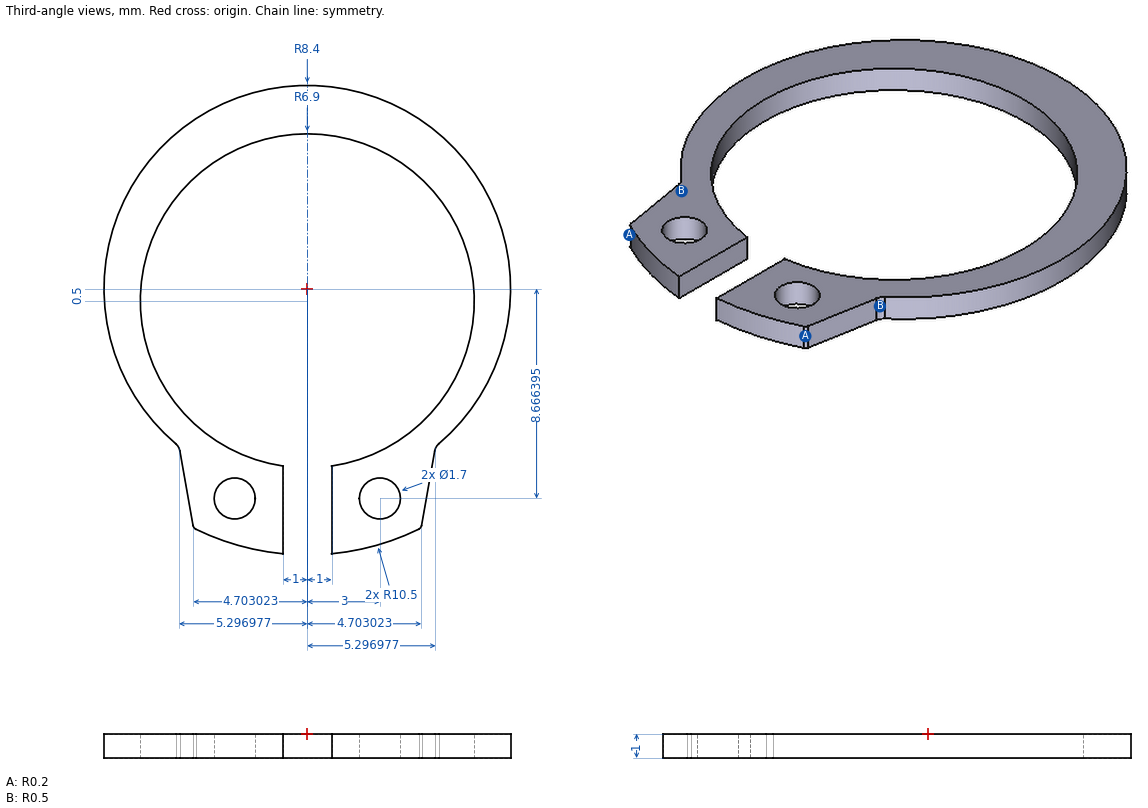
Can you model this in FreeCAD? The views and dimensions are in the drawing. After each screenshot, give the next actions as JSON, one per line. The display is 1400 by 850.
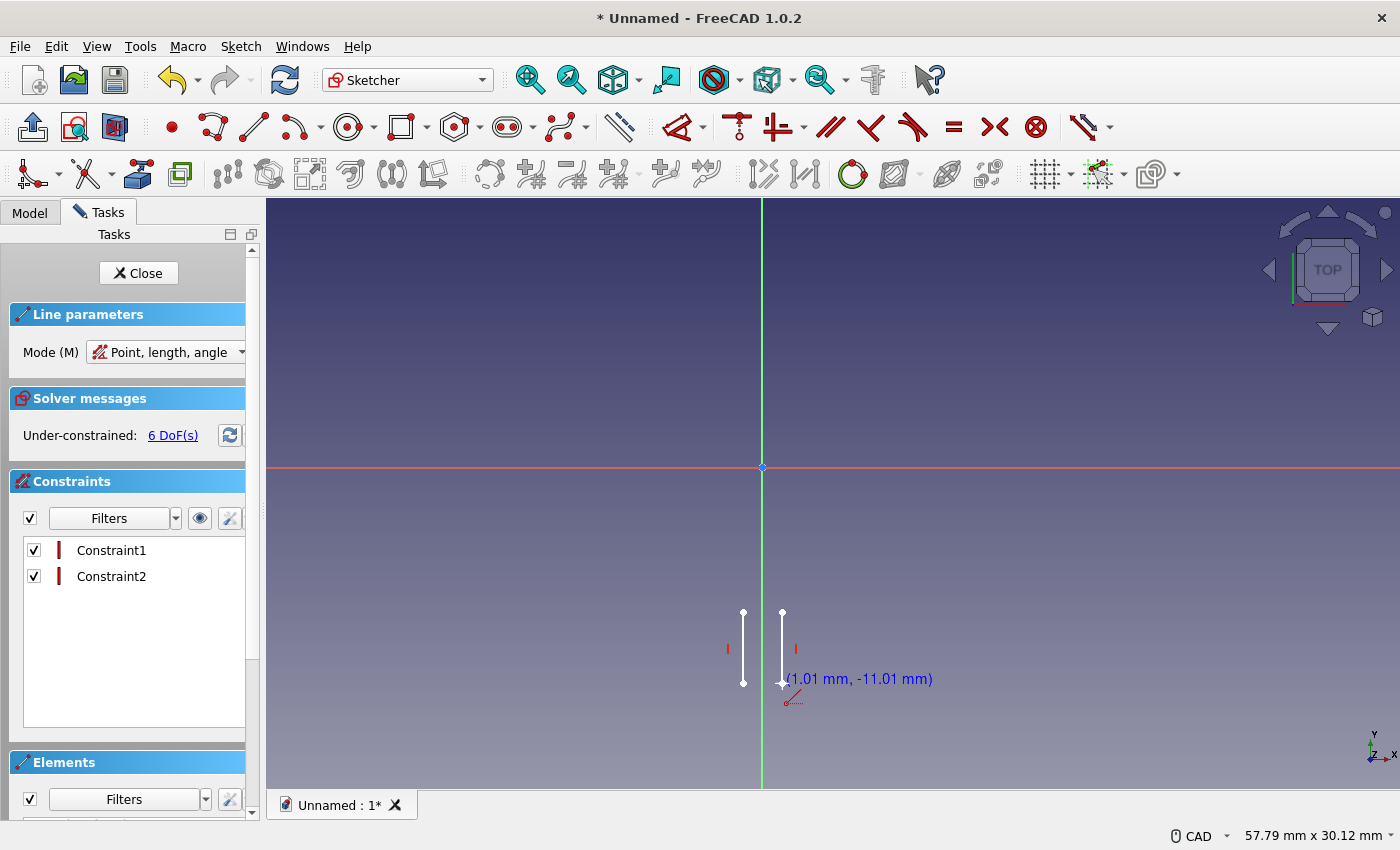
{"action": "left_click", "coordinate": [854, 662]}
{"action": "left_click", "coordinate": [866, 596]}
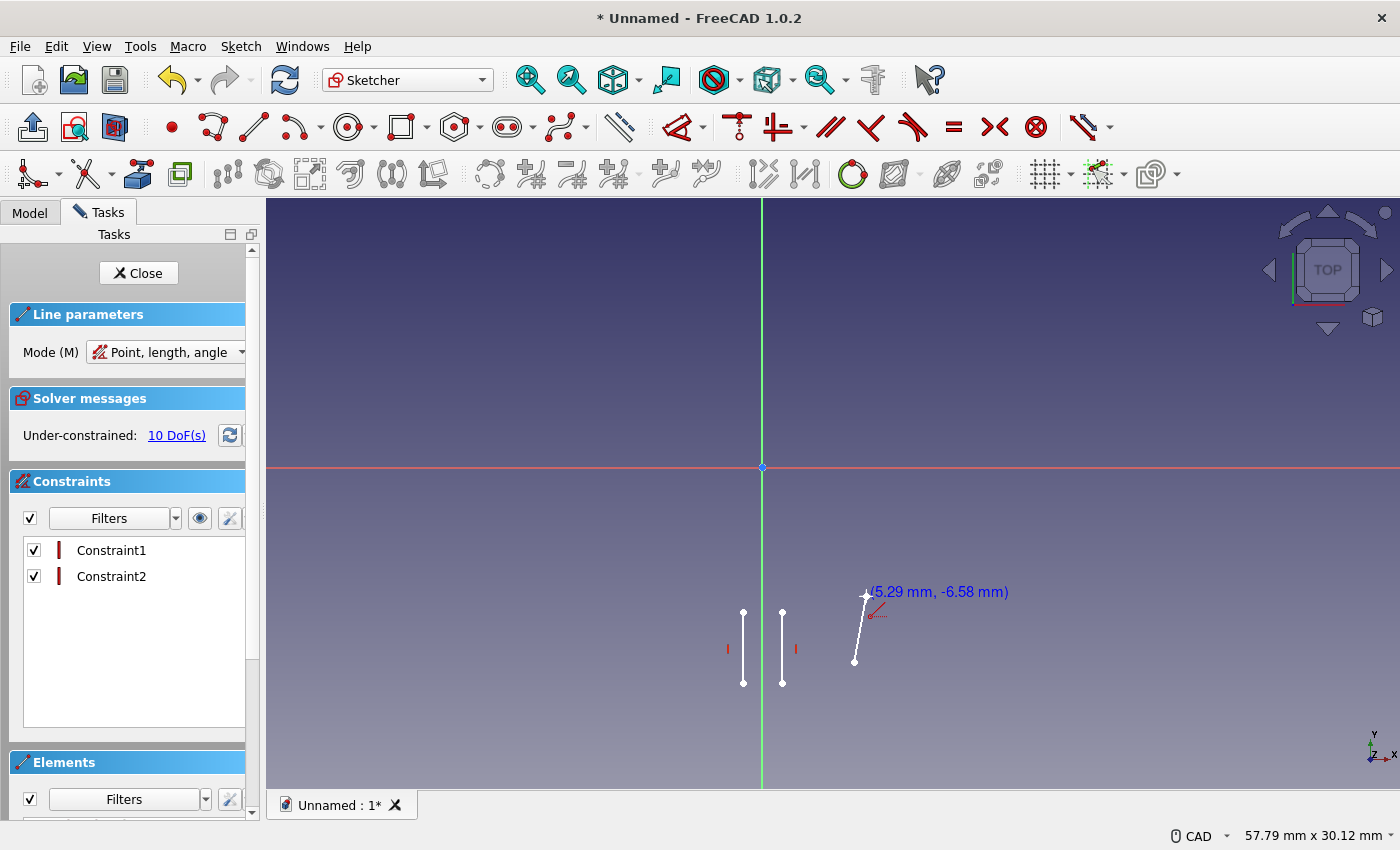
{"action": "left_click", "coordinate": [658, 596]}
{"action": "left_click", "coordinate": [670, 662]}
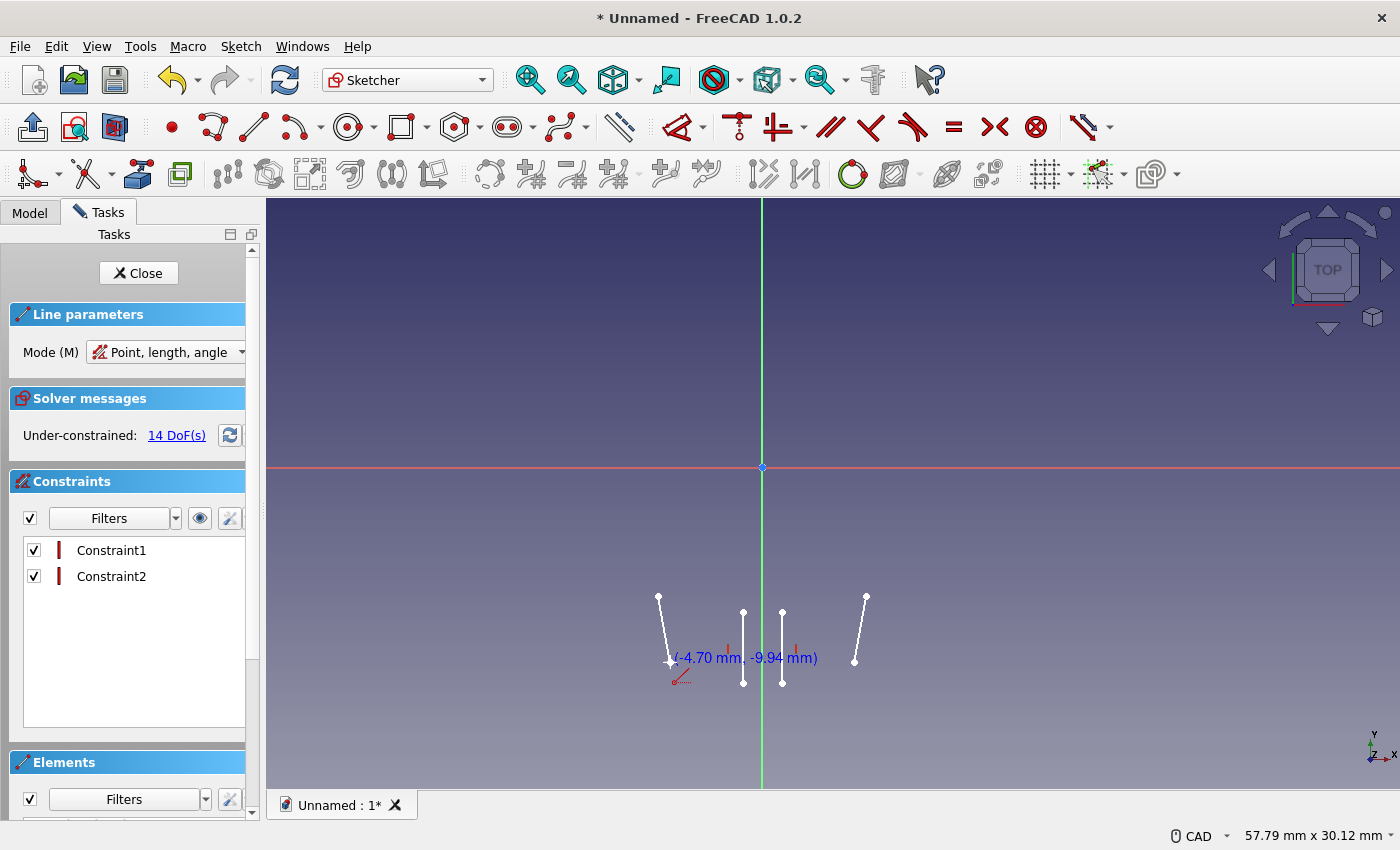
{"action": "left_click", "coordinate": [320, 128]}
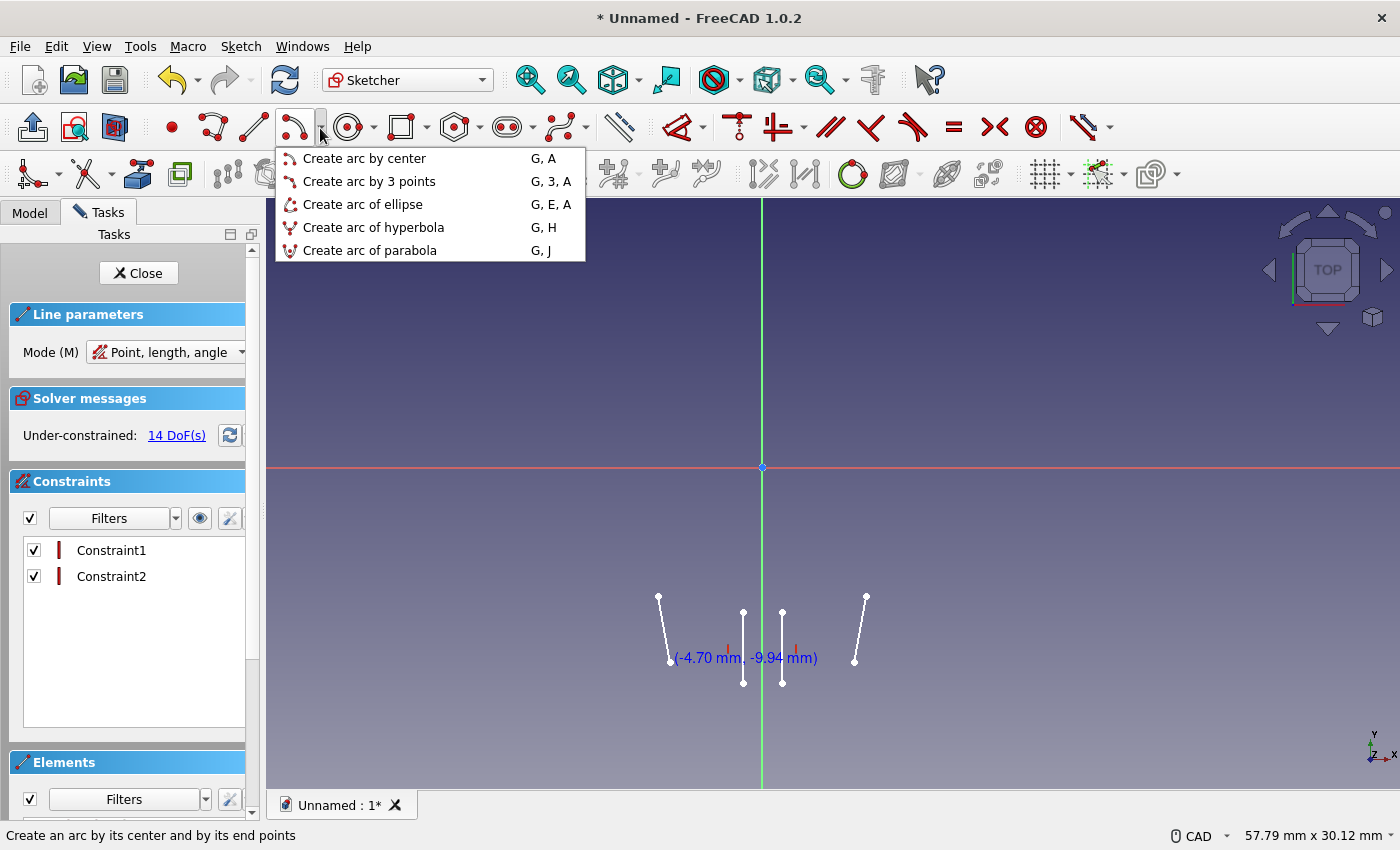
{"action": "left_click", "coordinate": [430, 182]}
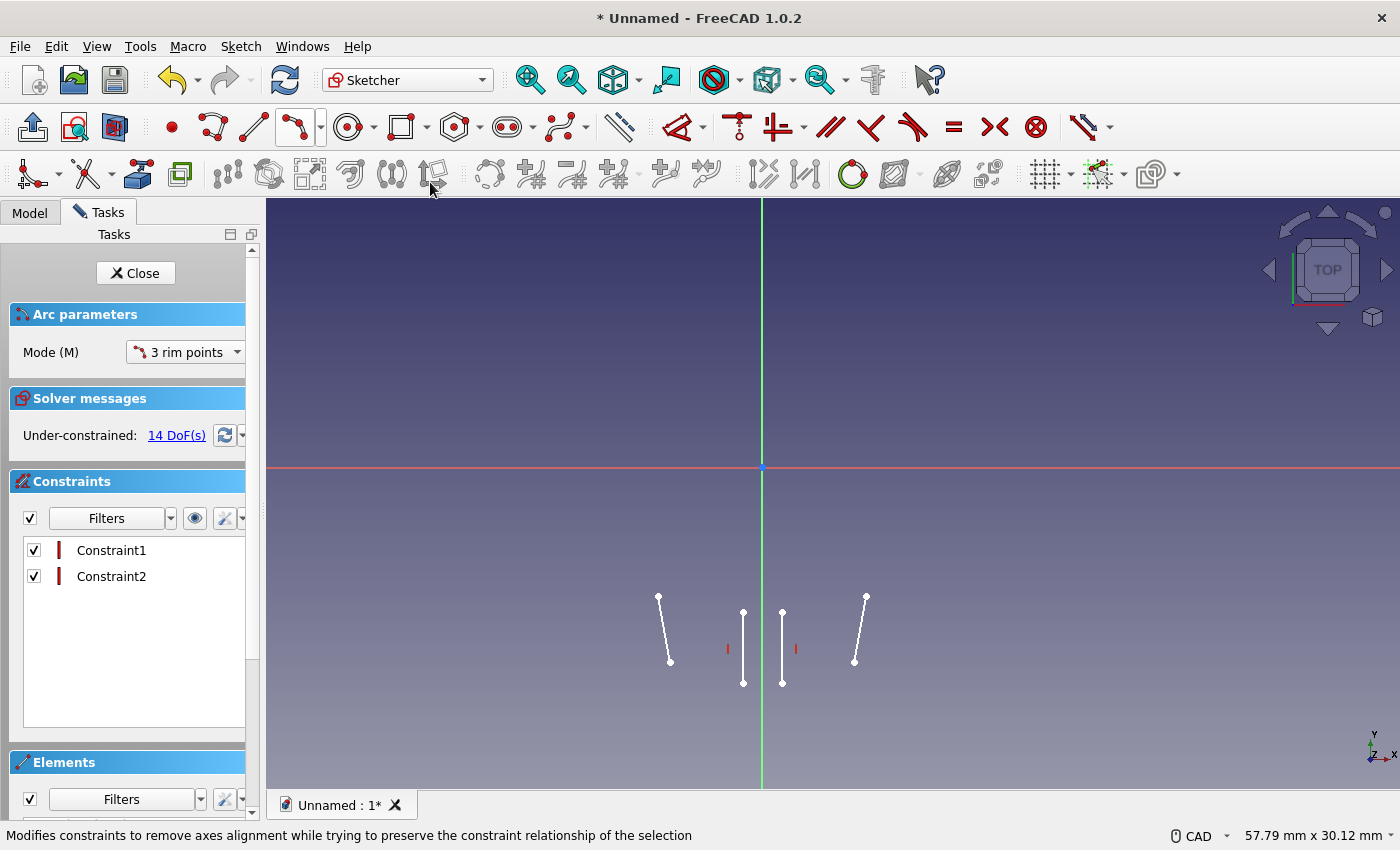
{"action": "left_click", "coordinate": [743, 613]}
{"action": "left_click", "coordinate": [782, 613]}
{"action": "left_click", "coordinate": [839, 366]}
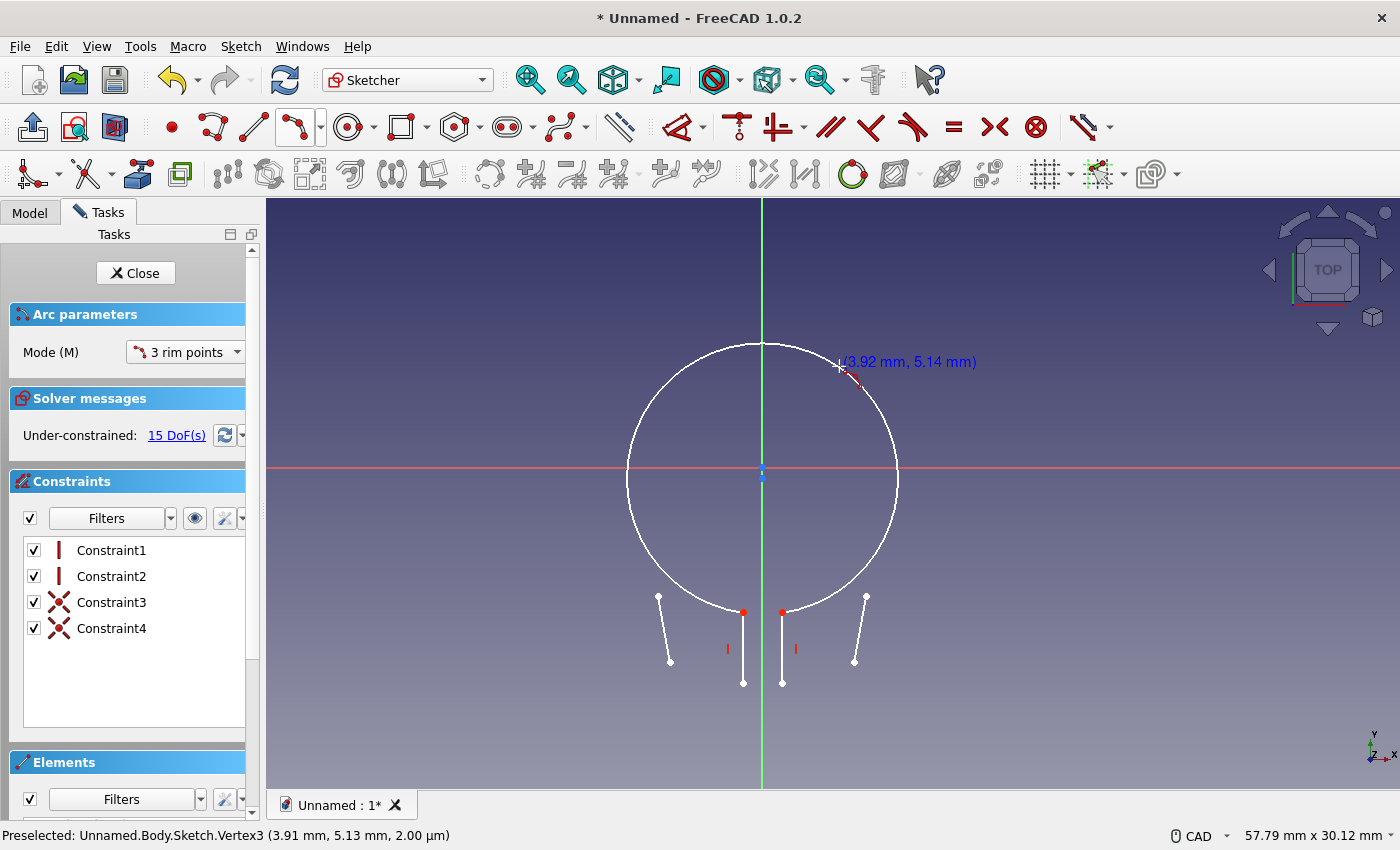
{"action": "left_click", "coordinate": [782, 684]}
{"action": "left_click", "coordinate": [854, 663]}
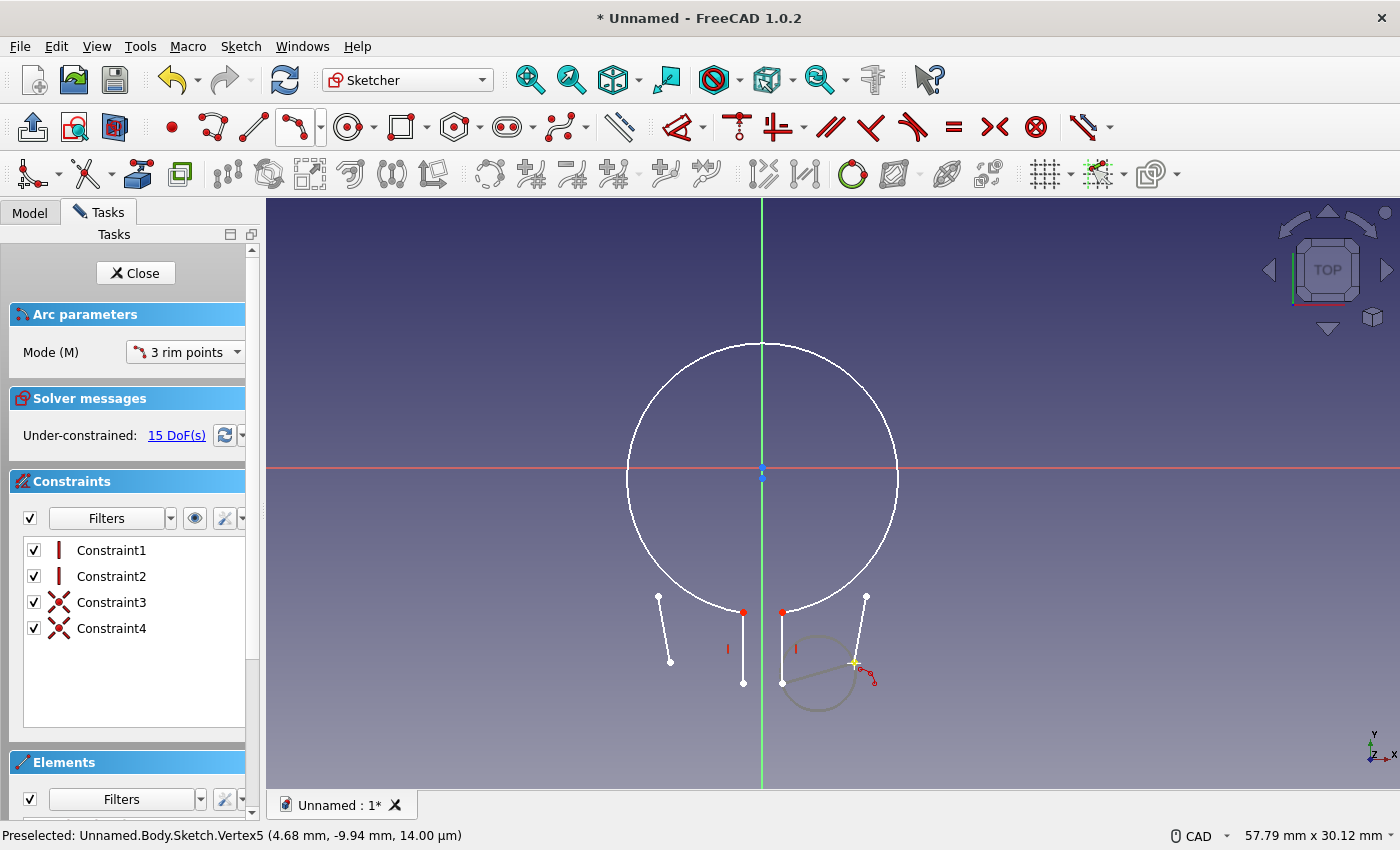
{"action": "scroll", "coordinate": [819, 676], "scroll_direction": "up", "scroll_amount": 8}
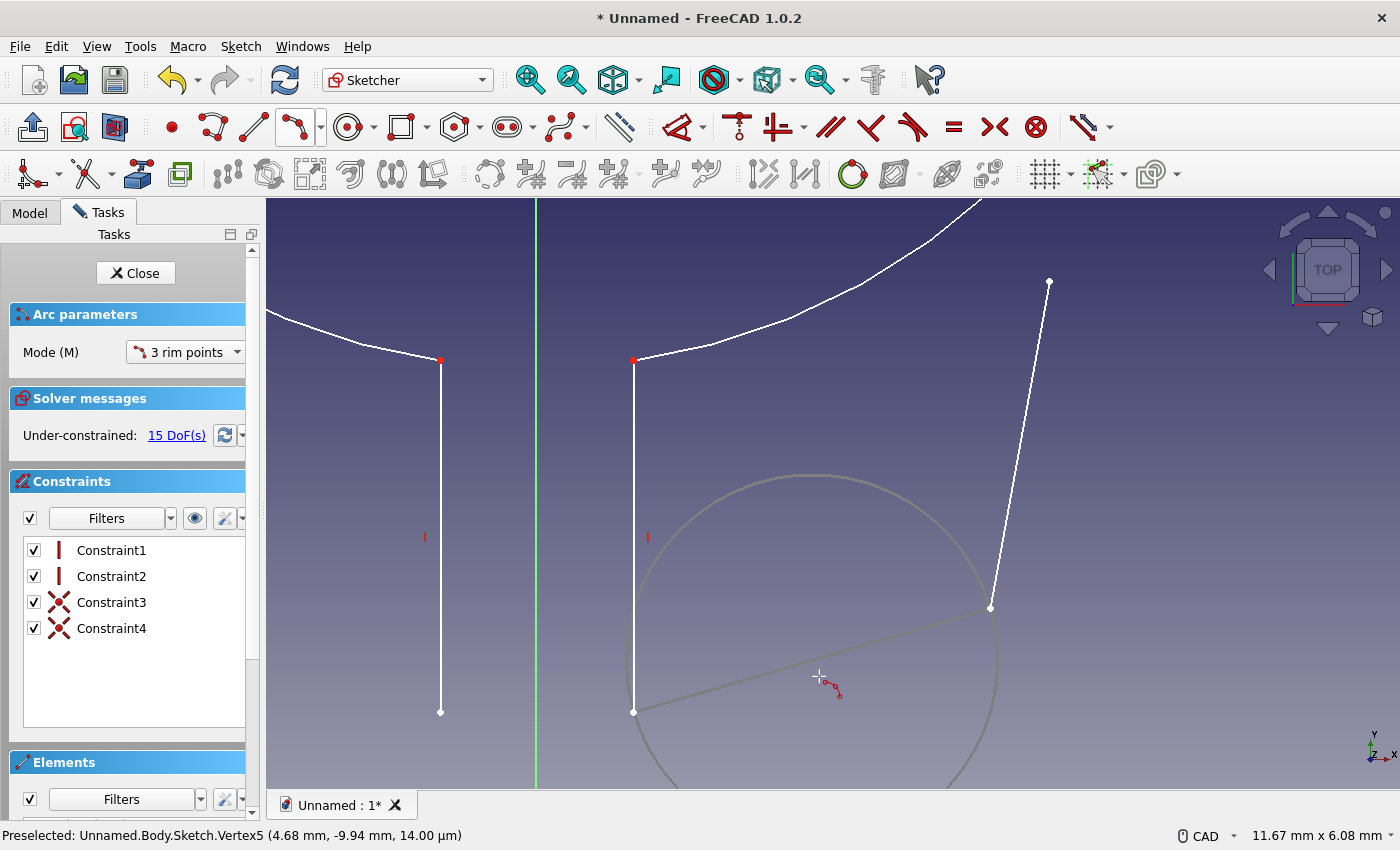
{"action": "left_click", "coordinate": [818, 672]}